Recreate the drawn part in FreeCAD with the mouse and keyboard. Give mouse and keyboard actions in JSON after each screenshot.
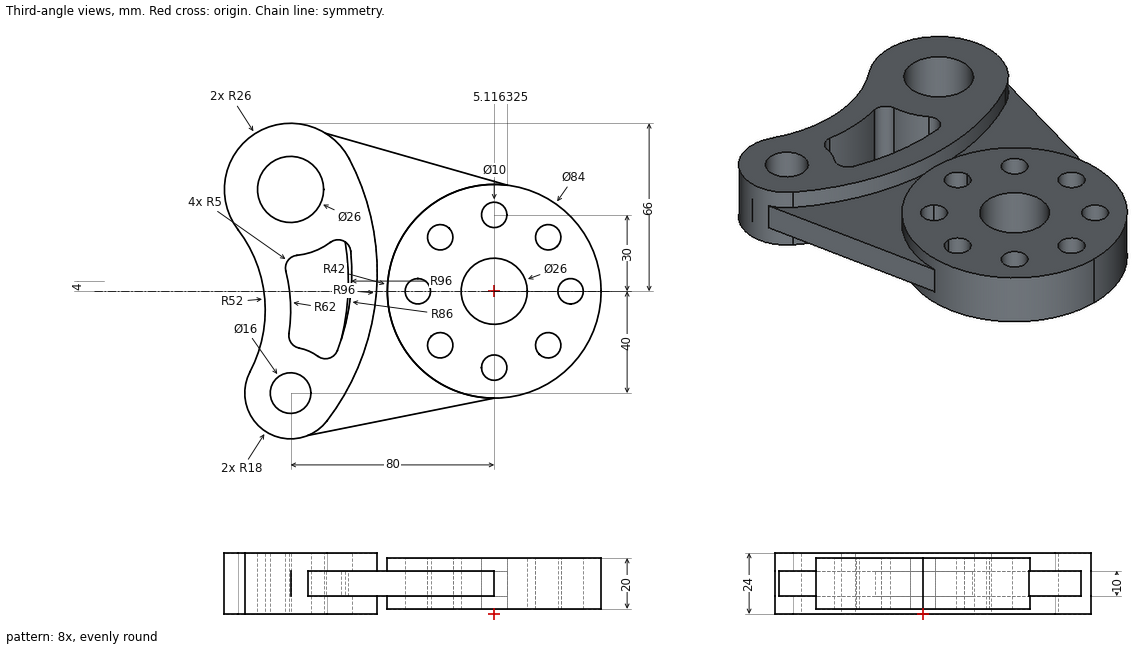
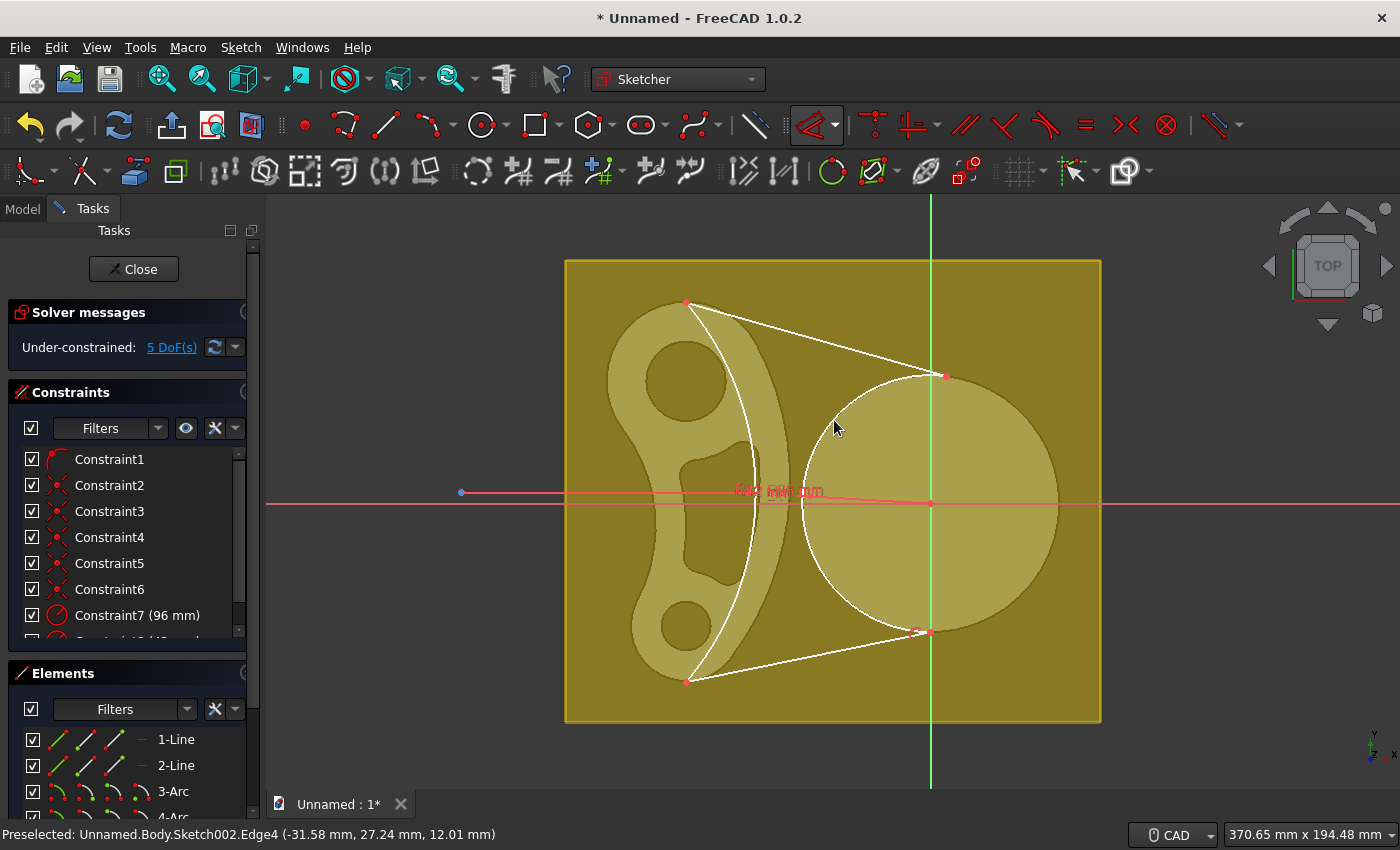
{"action": "scroll", "coordinate": [462, 492], "scroll_direction": "up", "scroll_amount": 6}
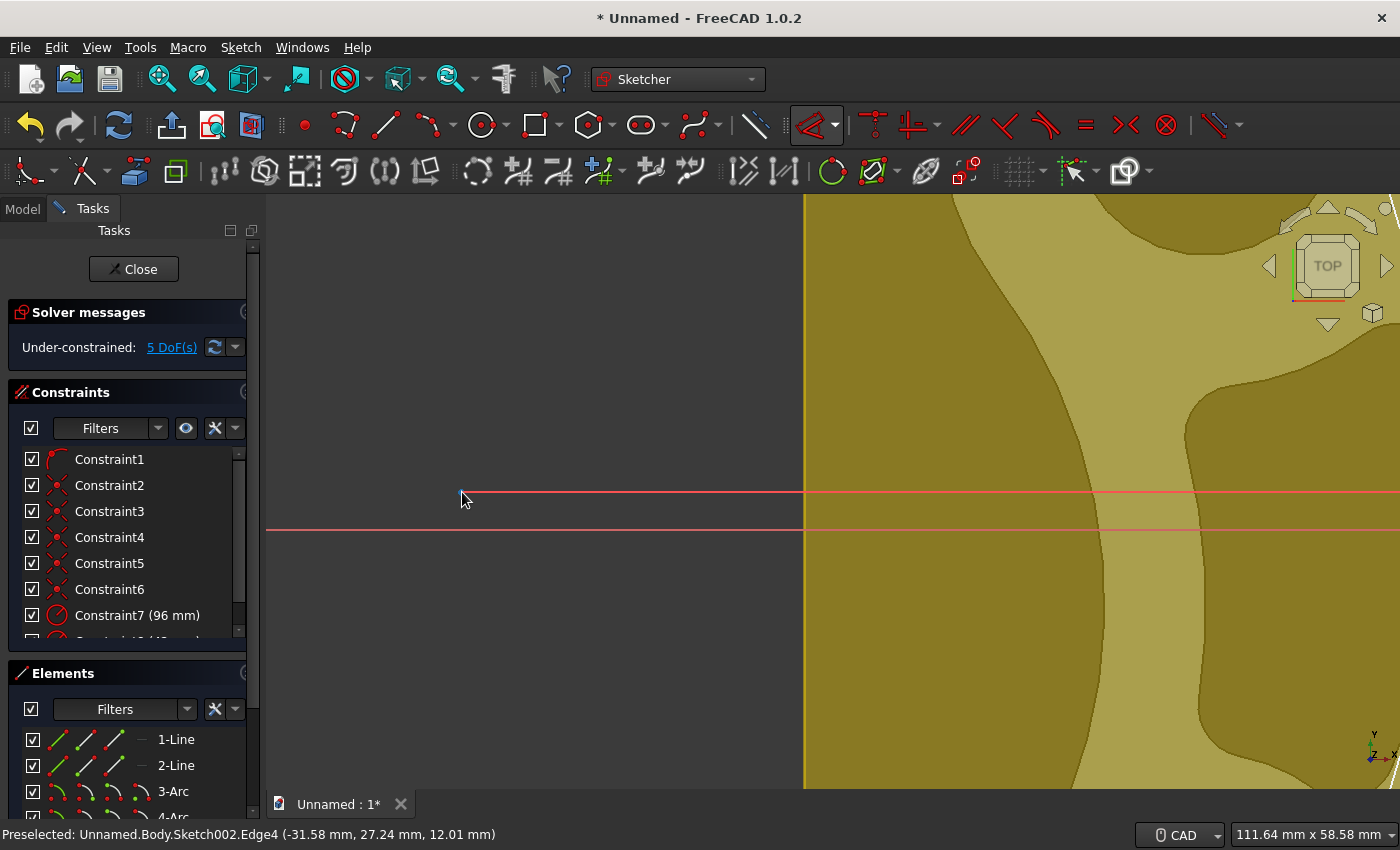
{"action": "left_click", "coordinate": [461, 492]}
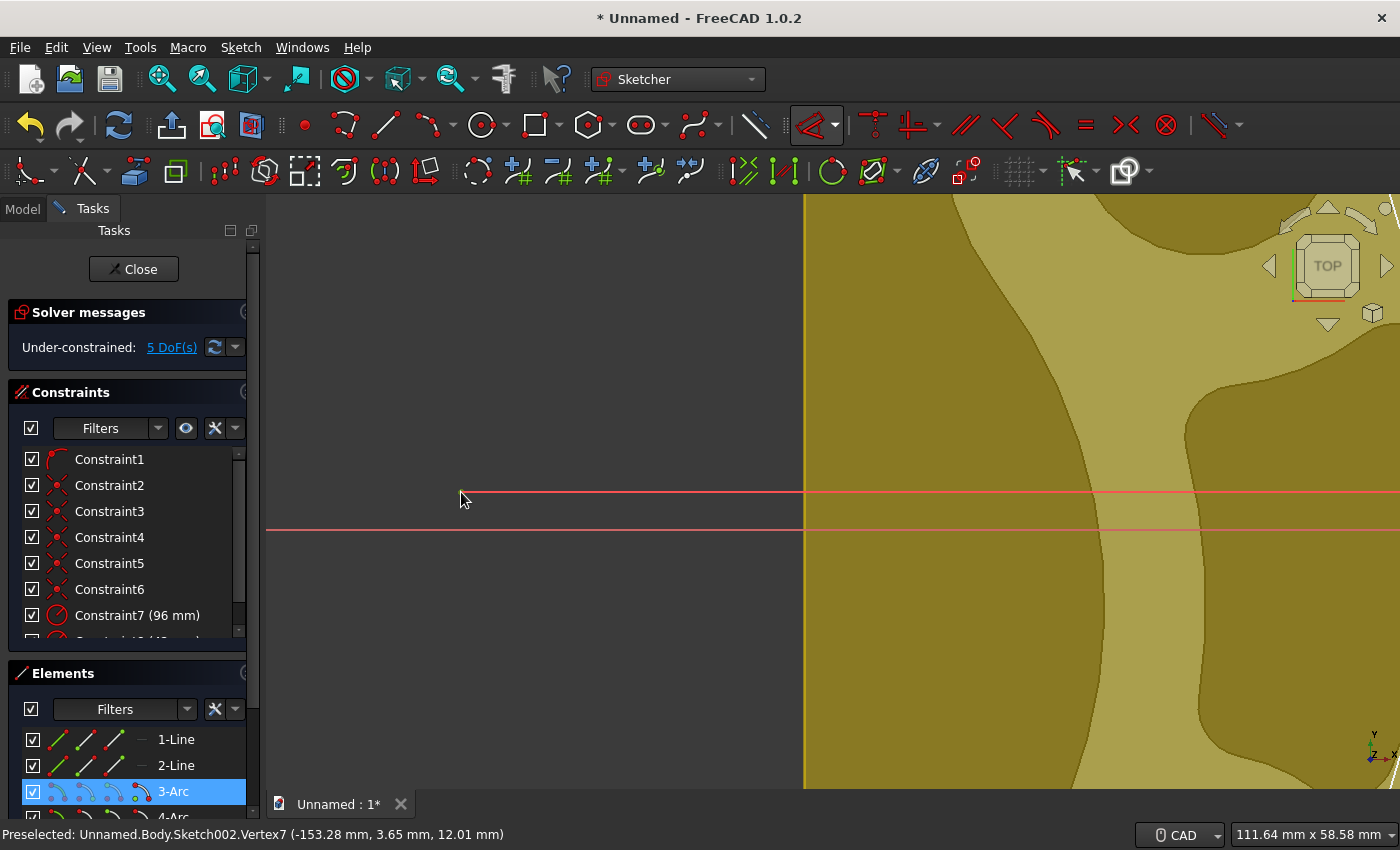
{"action": "left_click", "coordinate": [838, 126]}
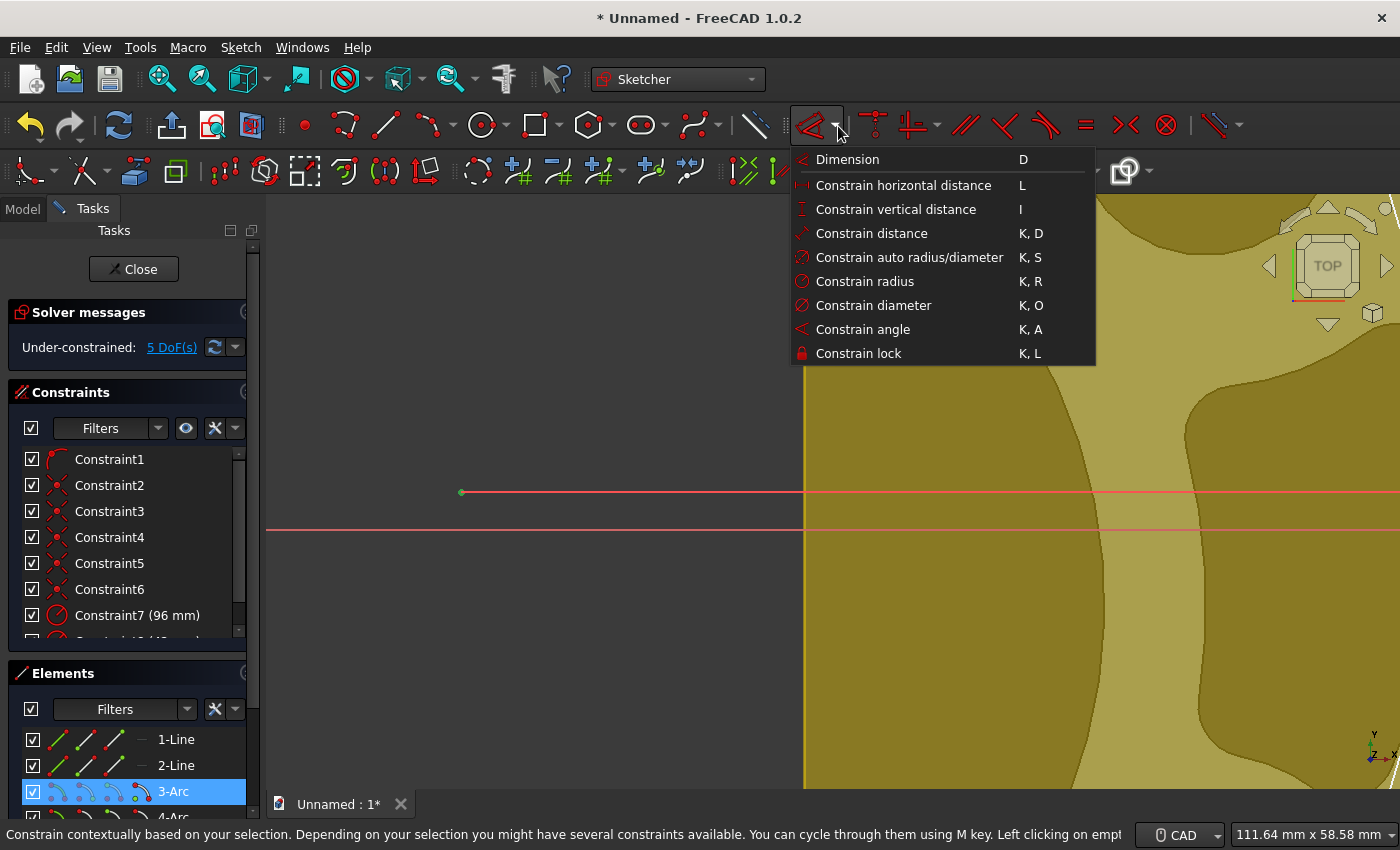
{"action": "left_click", "coordinate": [943, 209]}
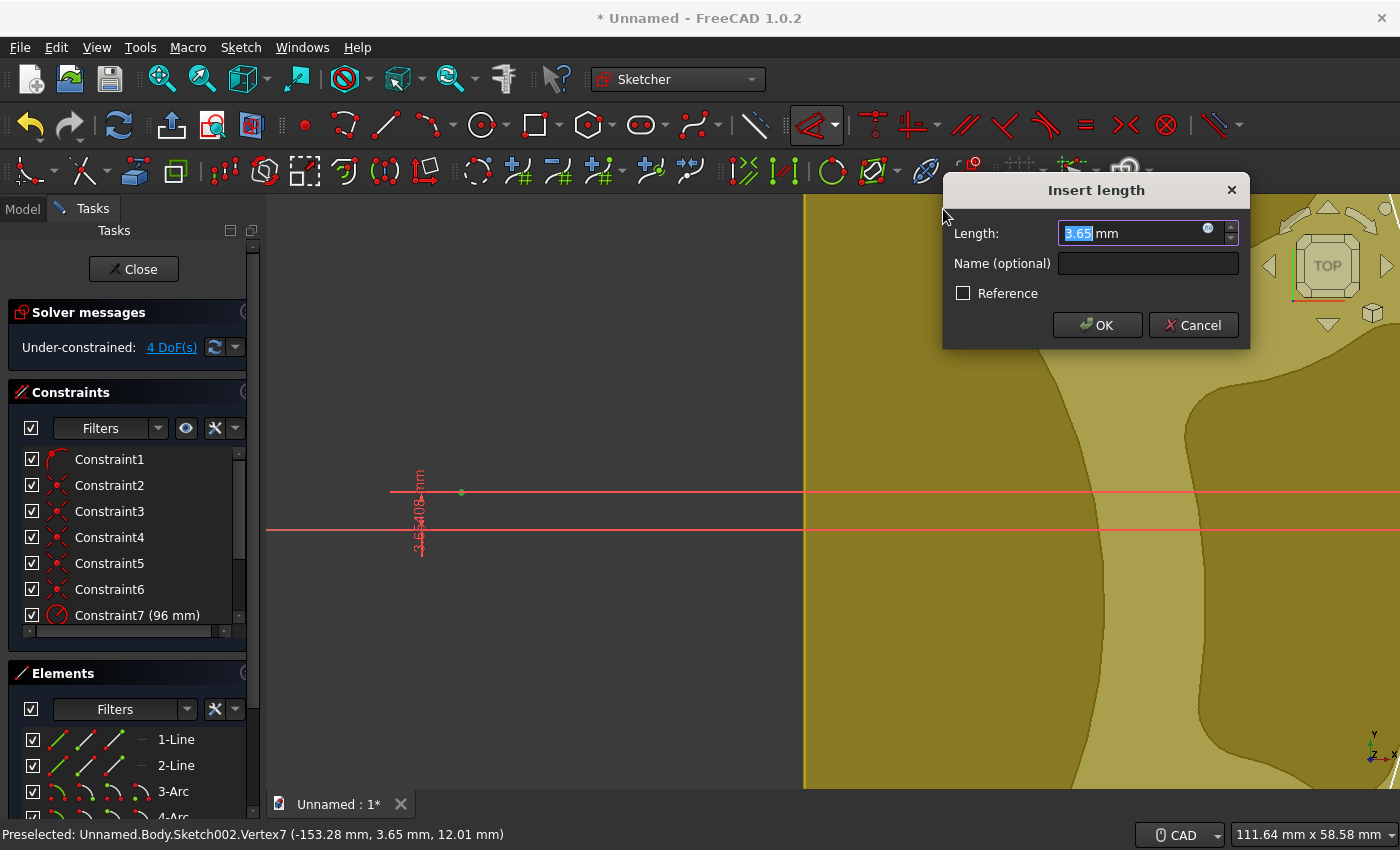
{"action": "type", "text": "4"}
{"action": "key", "text": "Return"}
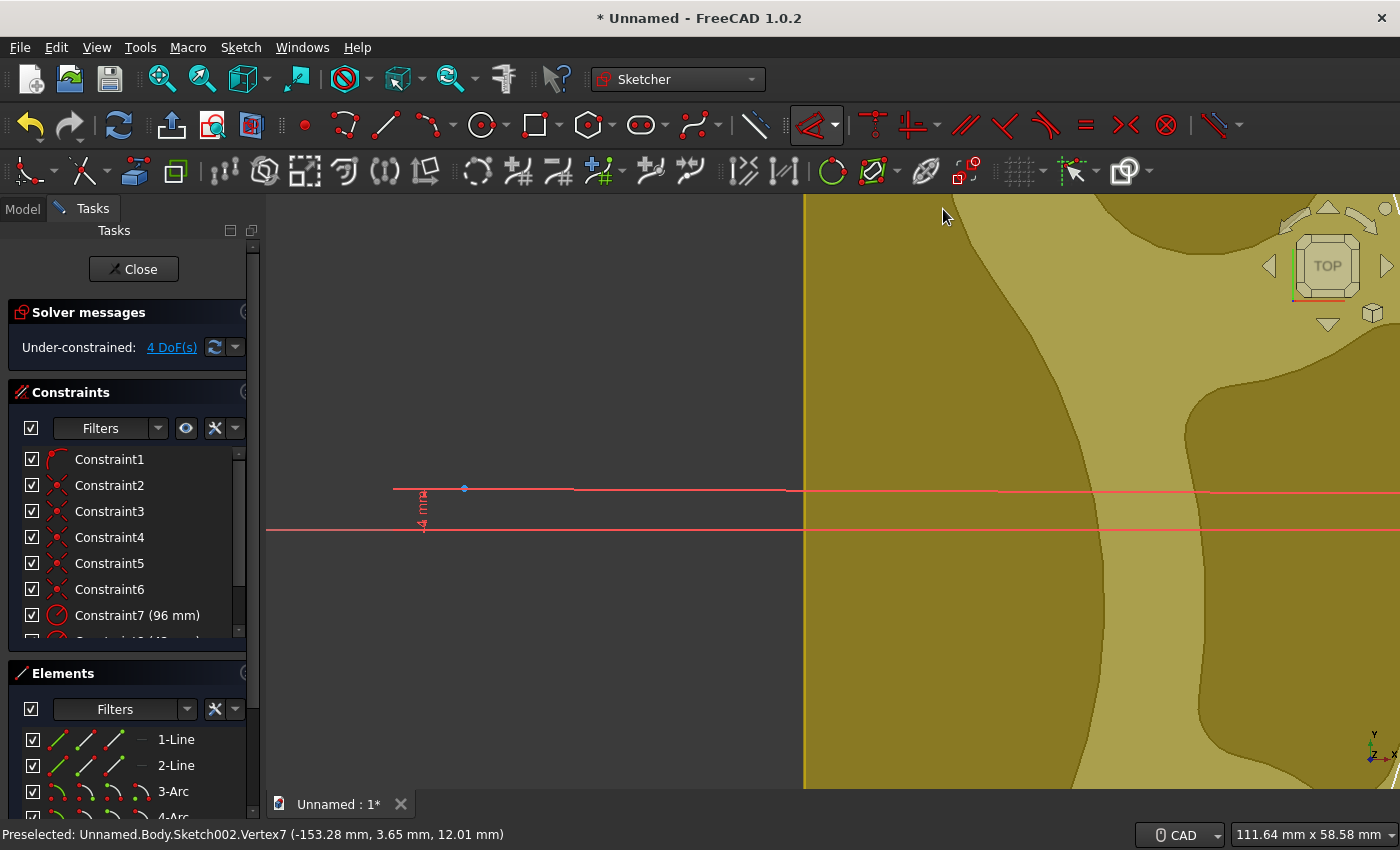
{"action": "scroll", "coordinate": [388, 493], "scroll_direction": "down", "scroll_amount": 6}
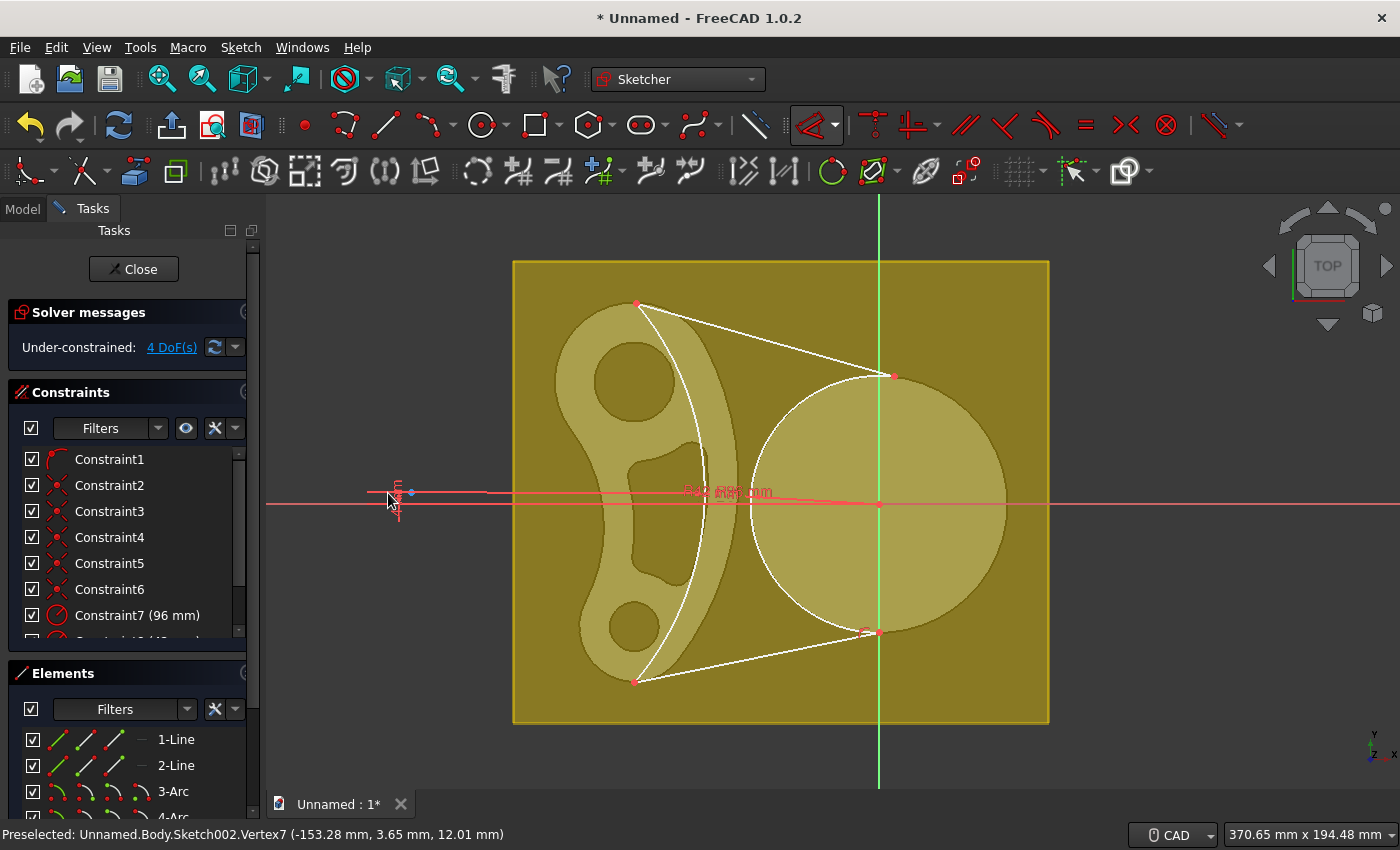
{"action": "left_click", "coordinate": [636, 304]}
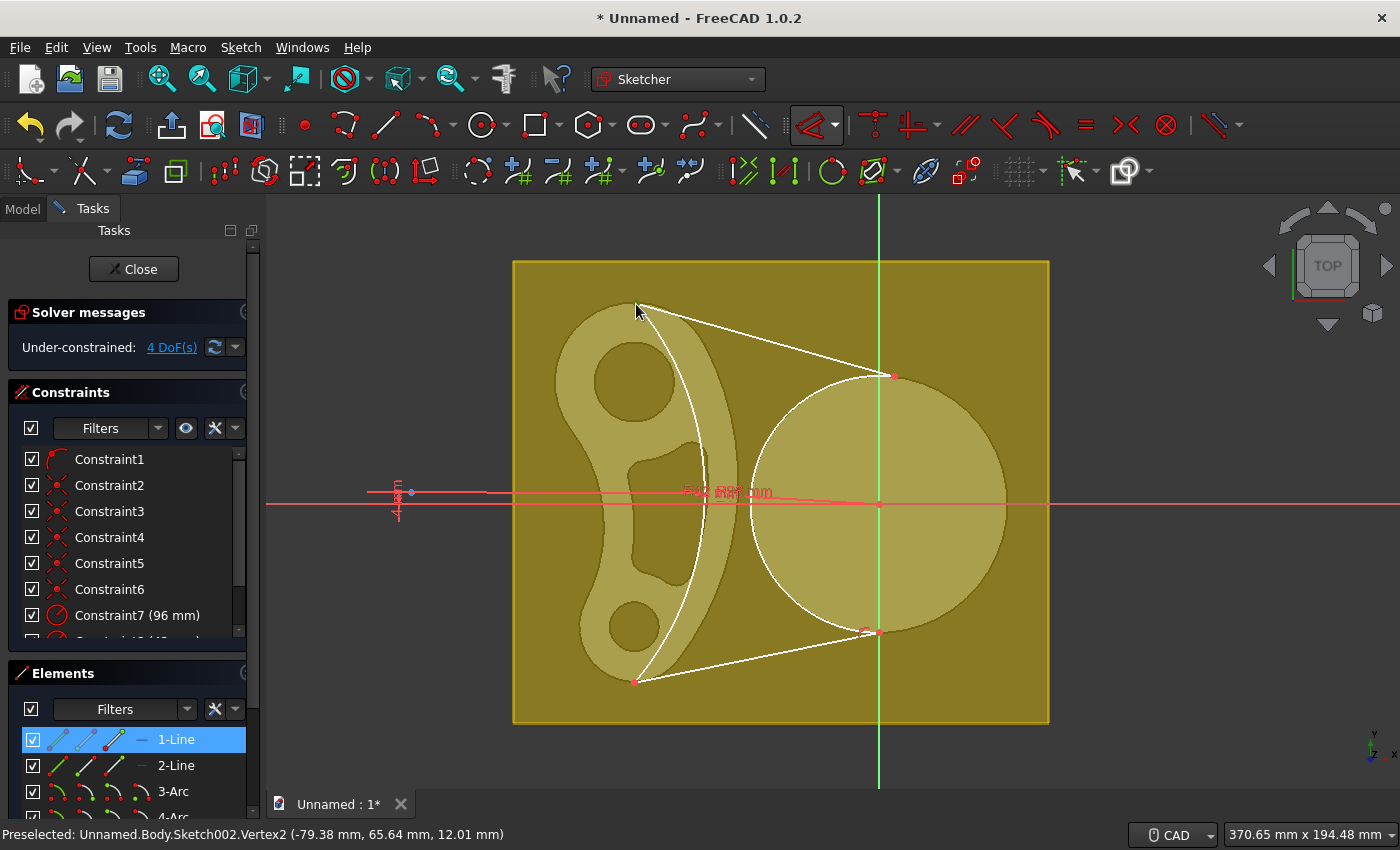
{"action": "key", "text": "l"}